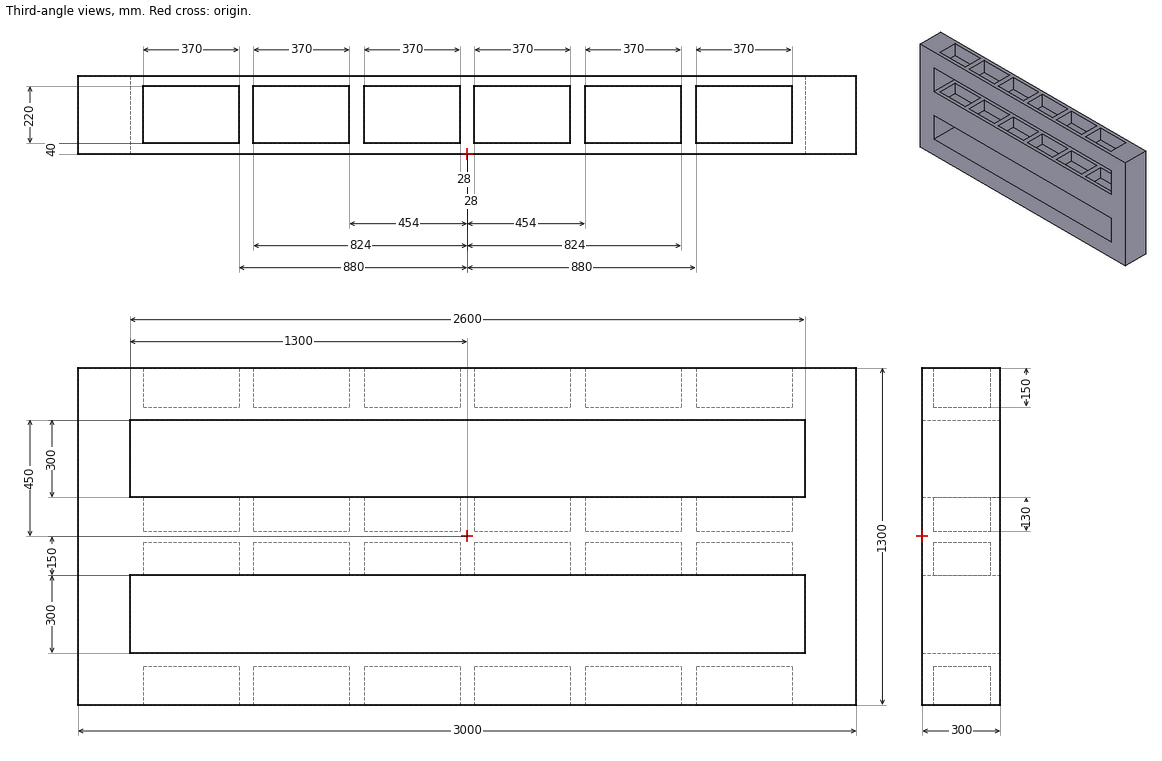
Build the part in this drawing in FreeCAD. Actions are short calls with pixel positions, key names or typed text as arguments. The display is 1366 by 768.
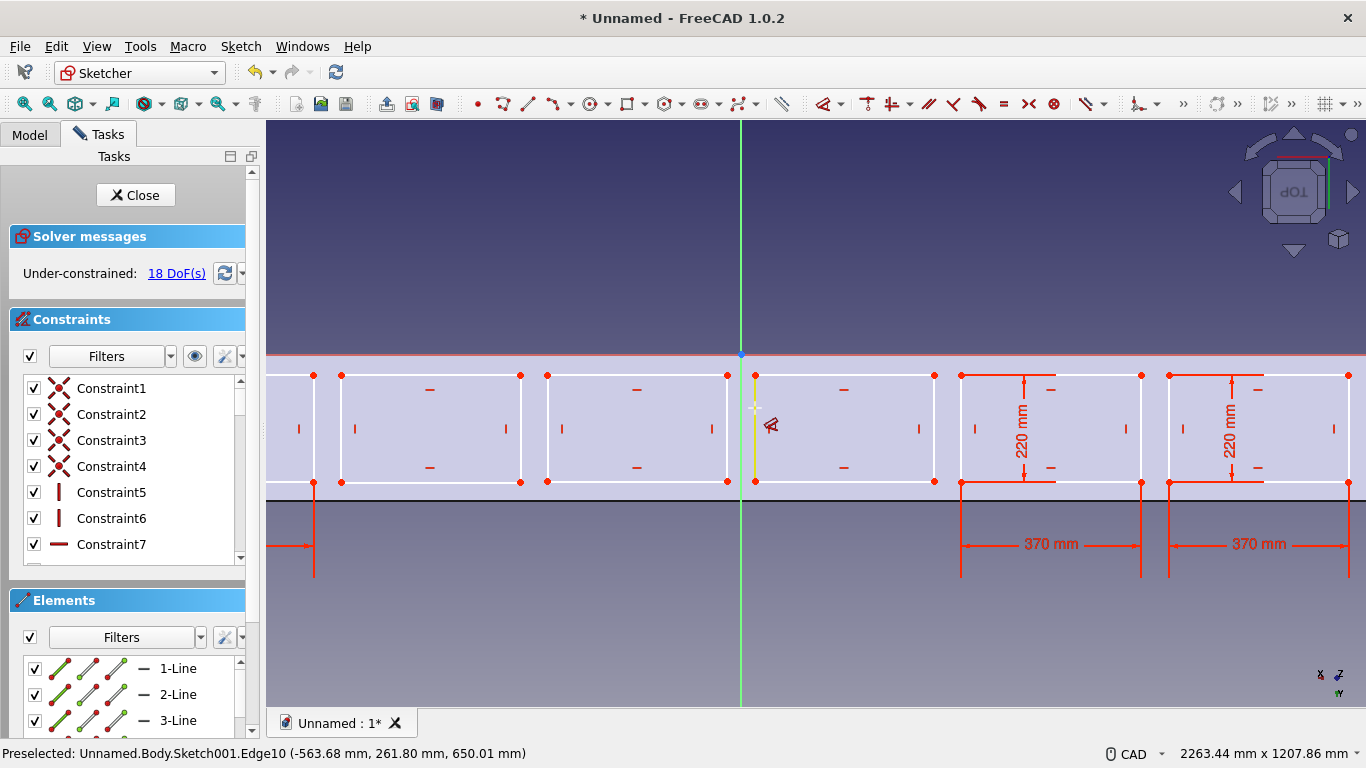
click(755, 407)
click(789, 428)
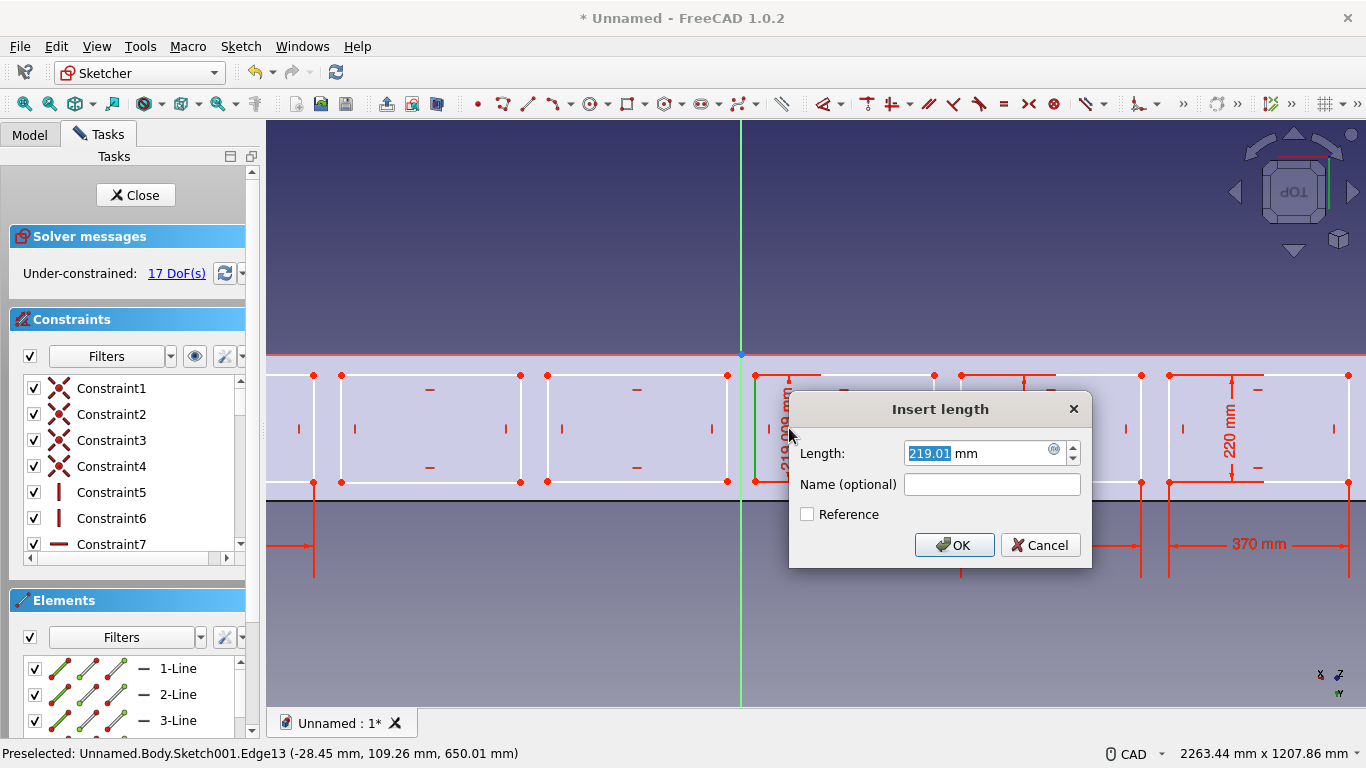
text(220)
key(Return)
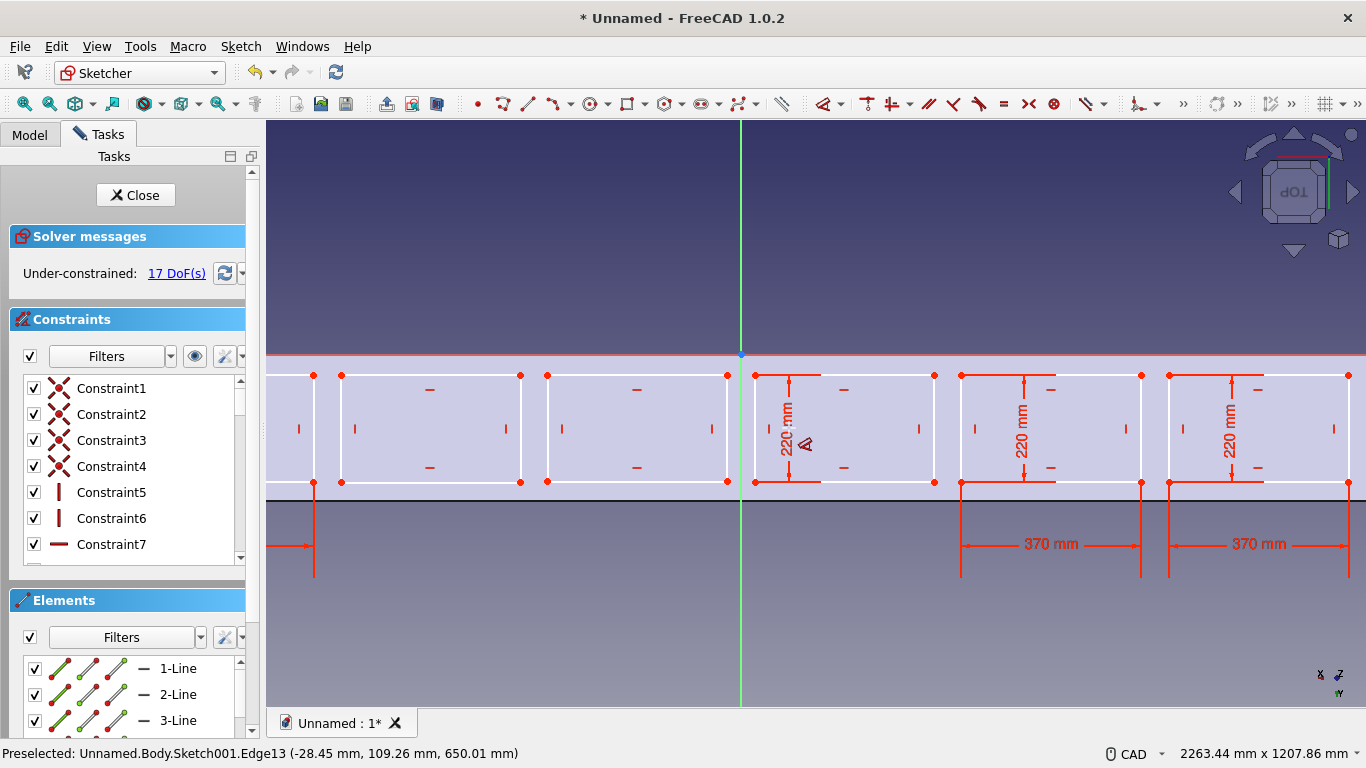
click(809, 482)
click(845, 516)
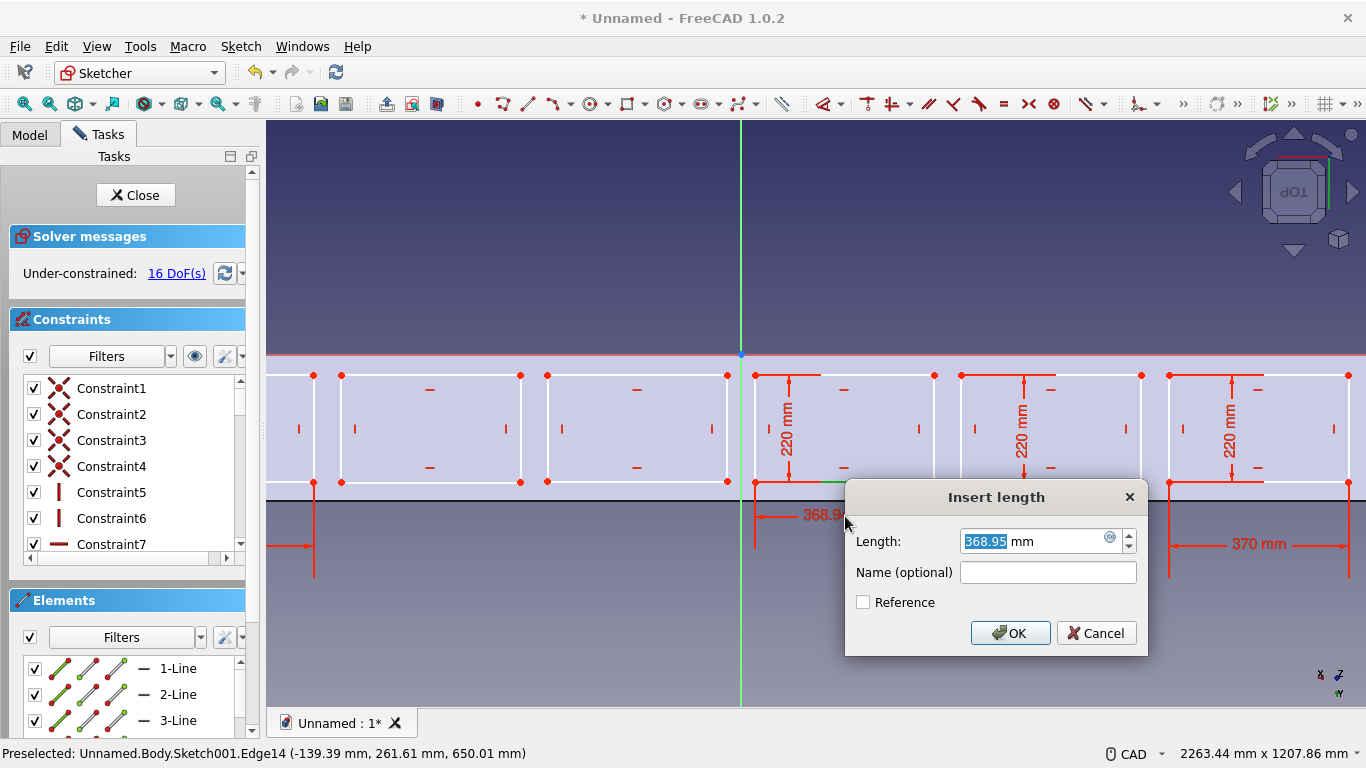
text(370)
key(Return)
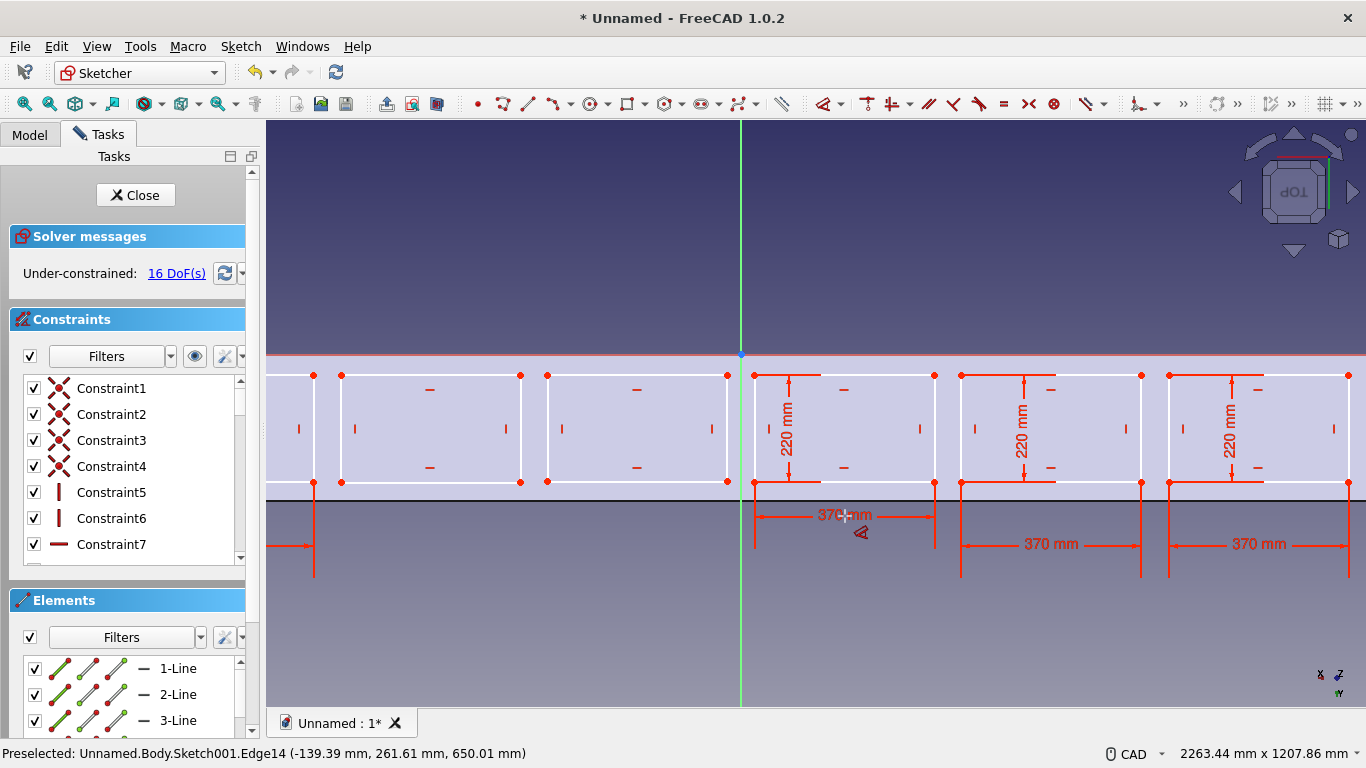
click(548, 407)
click(582, 428)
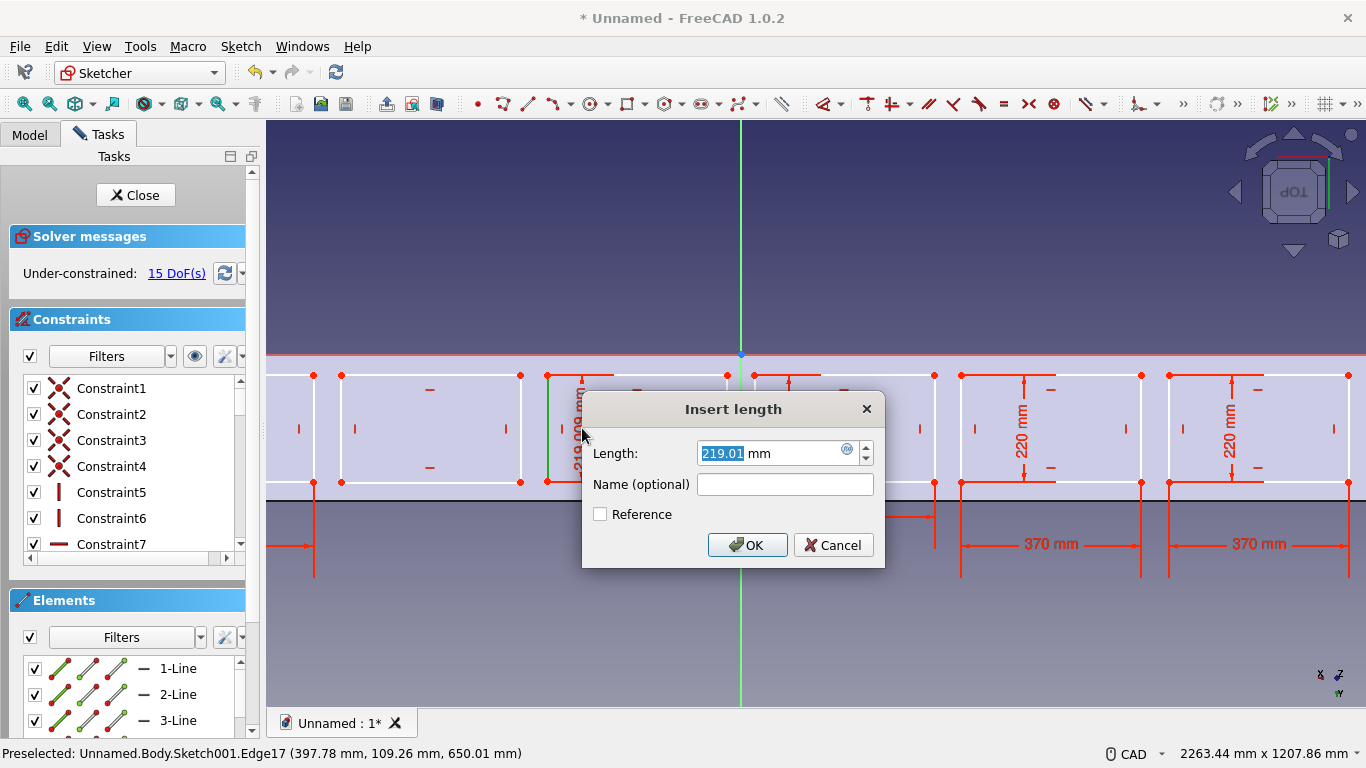
text(220)
key(Return)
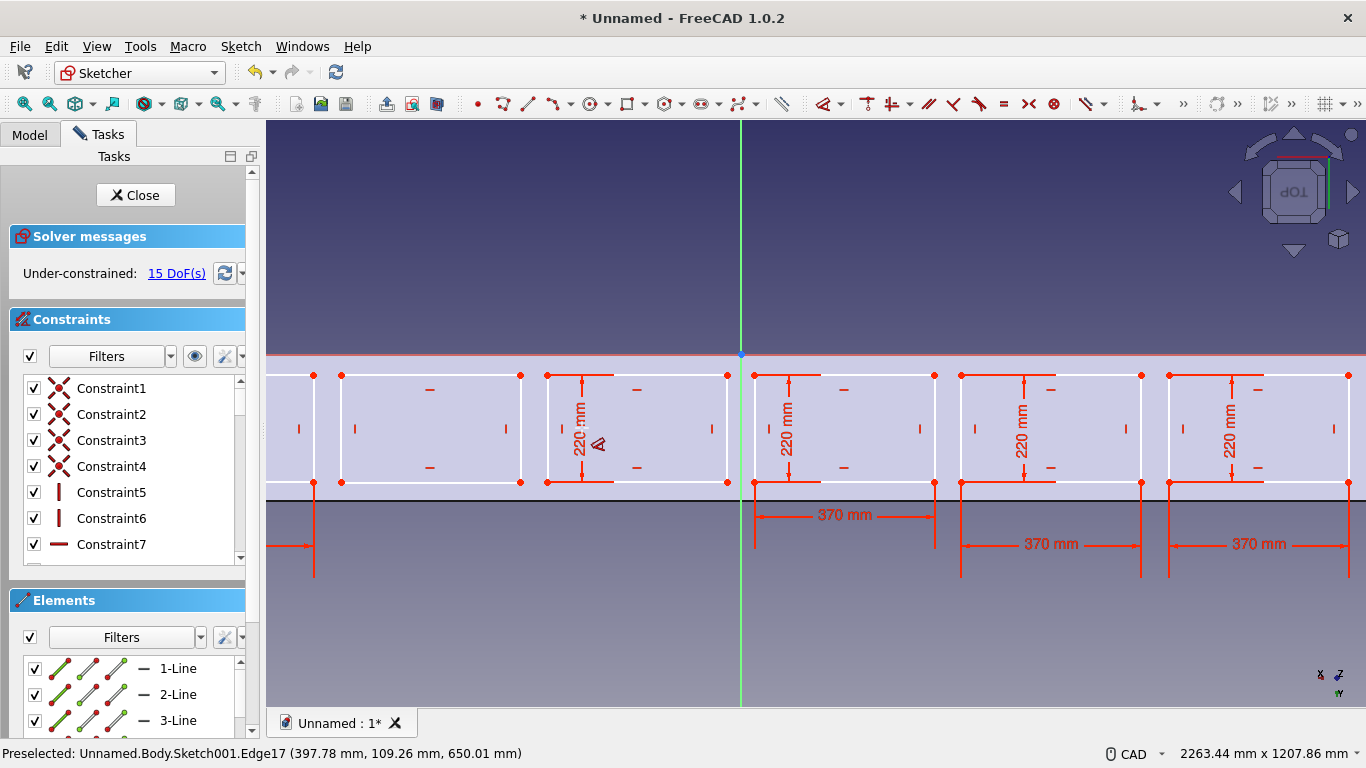
click(602, 482)
click(638, 516)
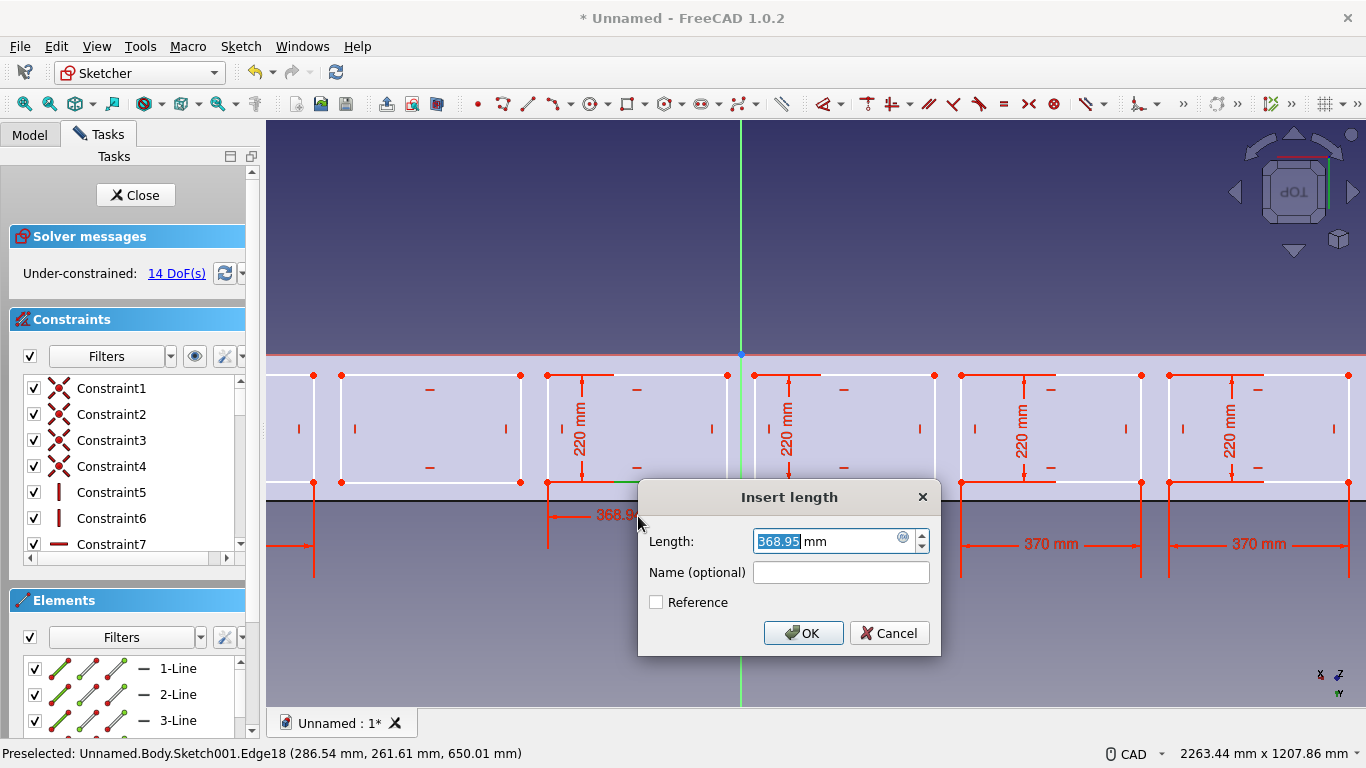
text(370)
key(Return)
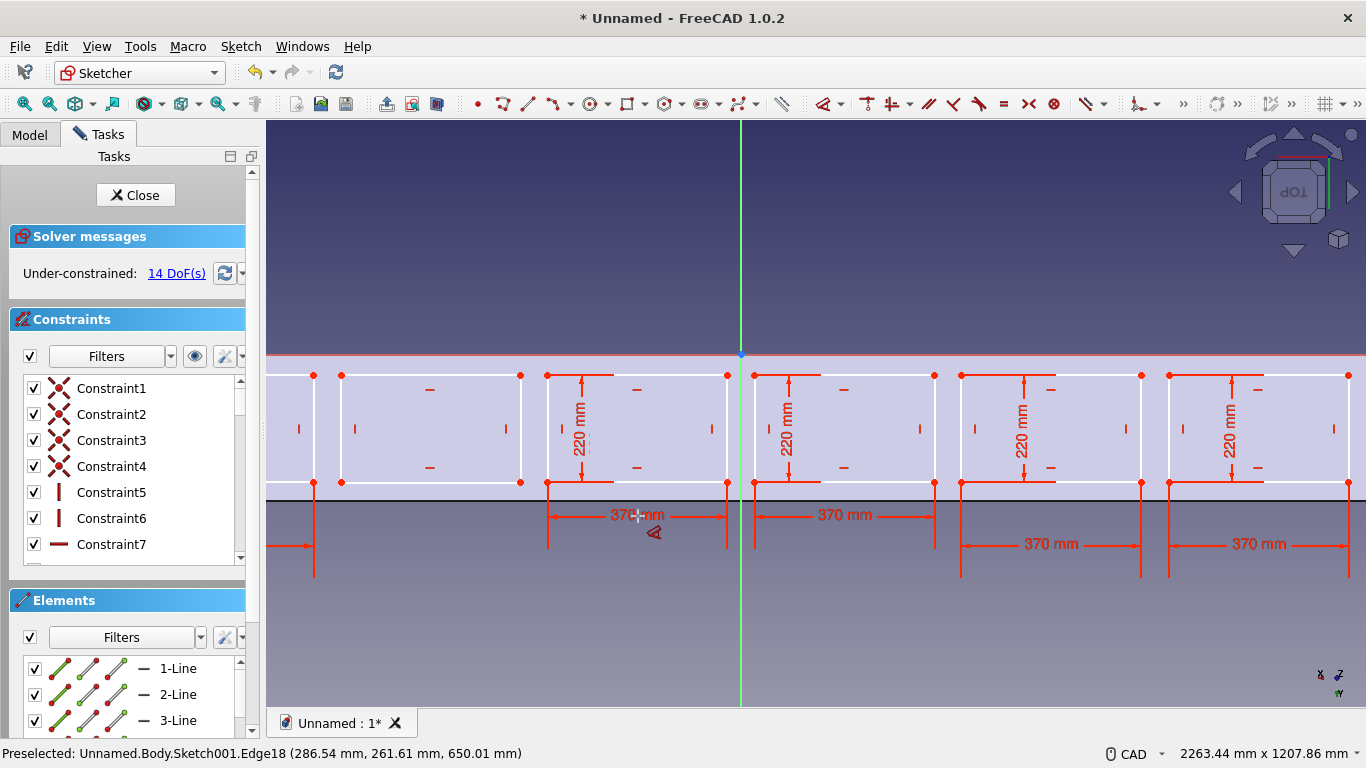
click(341, 407)
click(375, 429)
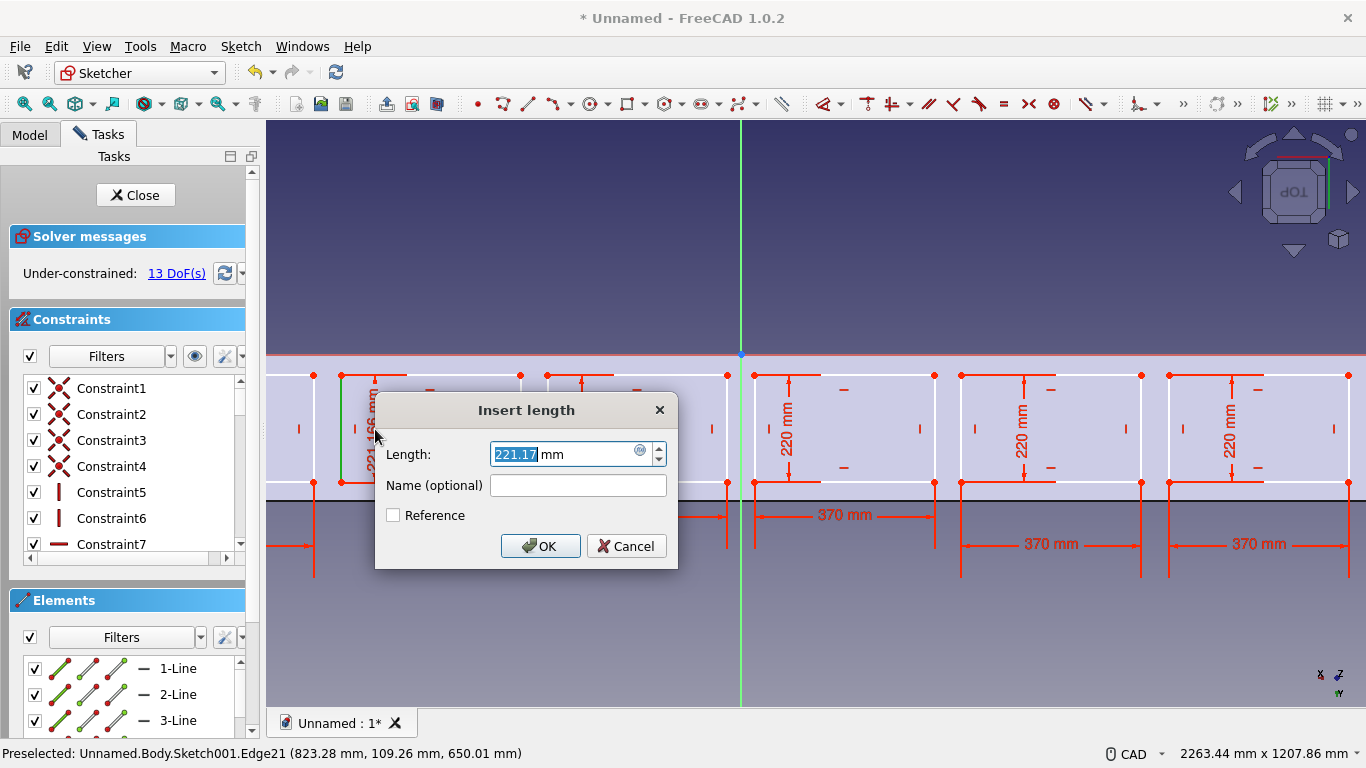
text(220)
key(Return)